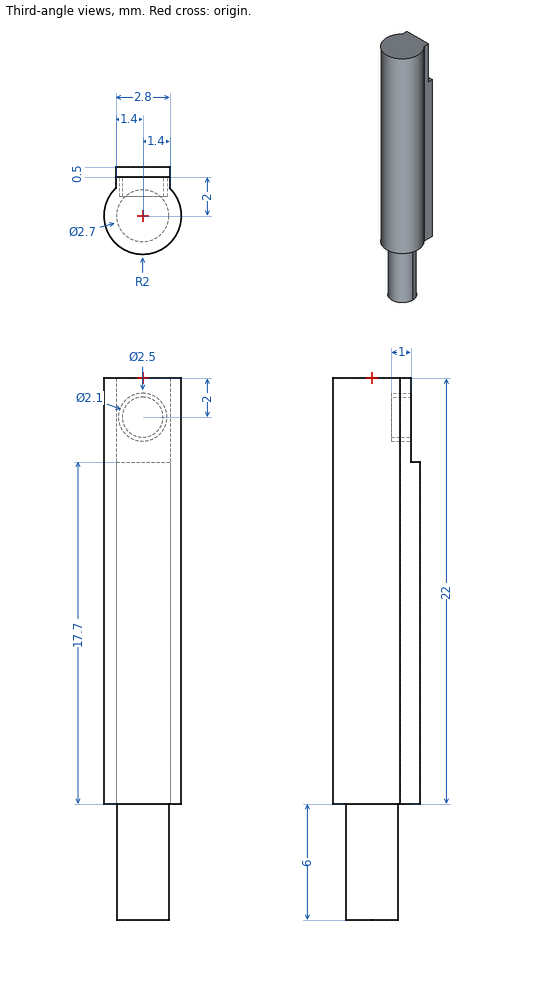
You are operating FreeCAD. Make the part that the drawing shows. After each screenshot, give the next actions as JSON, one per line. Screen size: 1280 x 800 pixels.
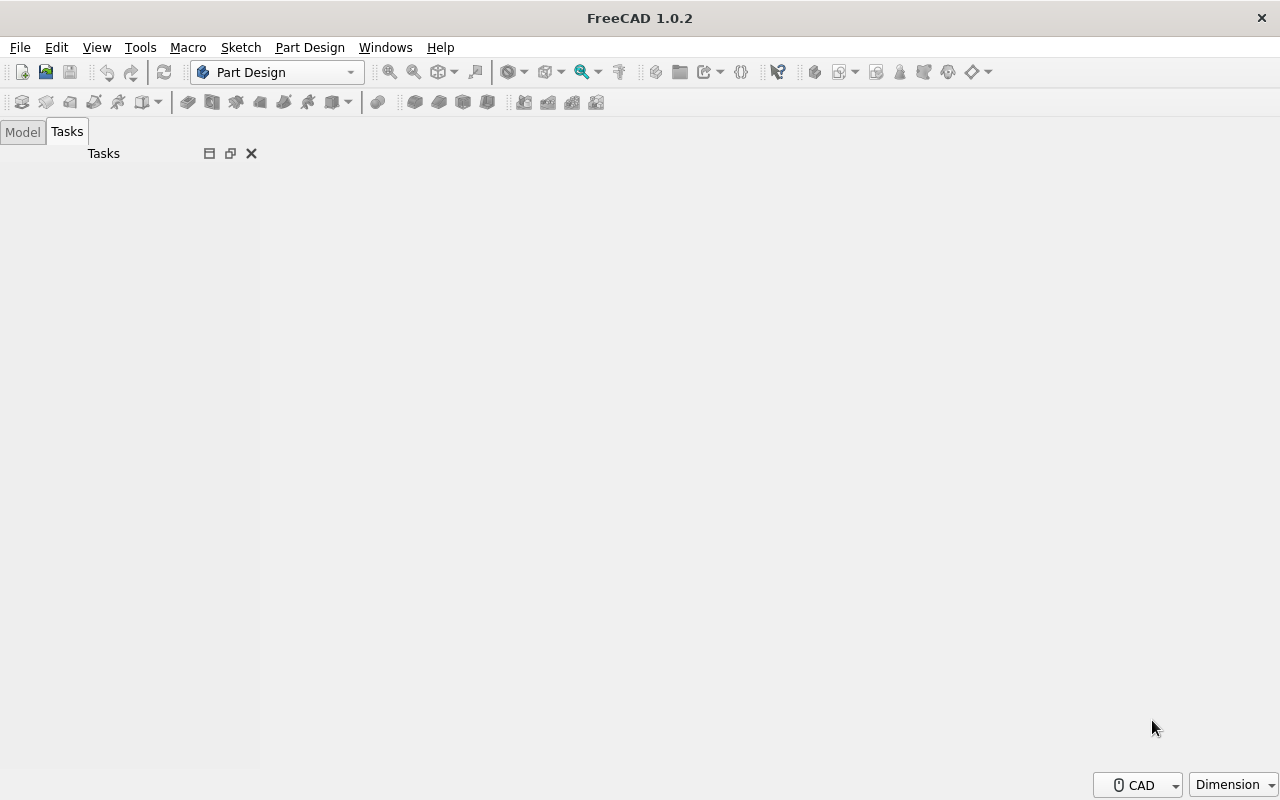
{"action": "key", "text": "ctrl+n"}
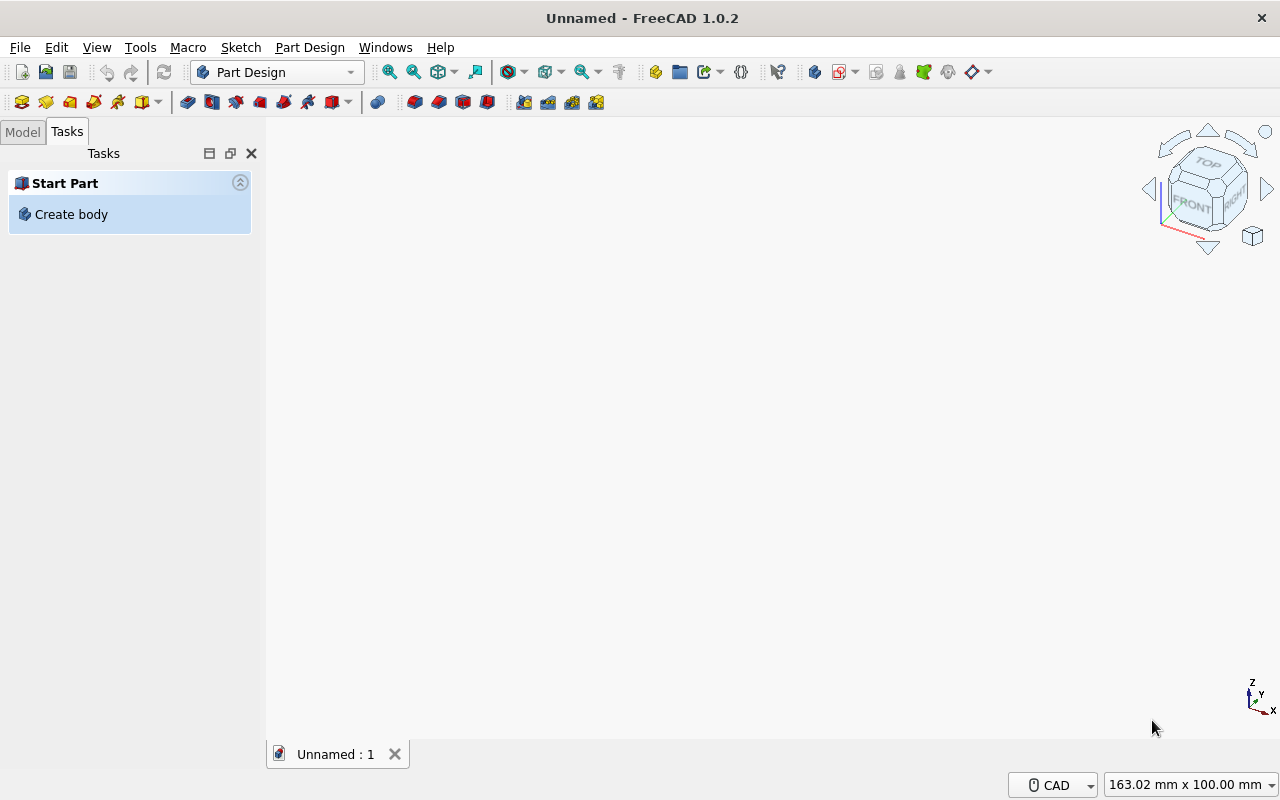
{"action": "left_click", "coordinate": [840, 72]}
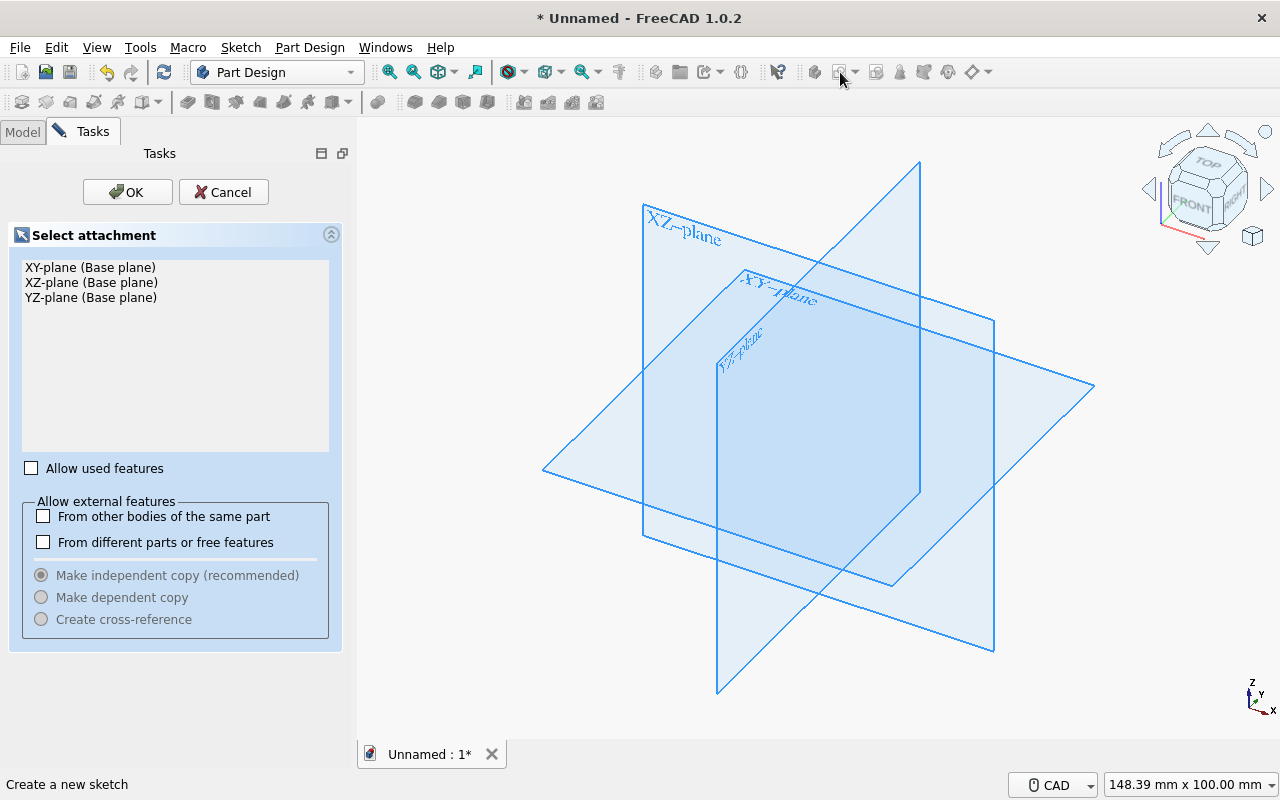
{"action": "left_click", "coordinate": [82, 268]}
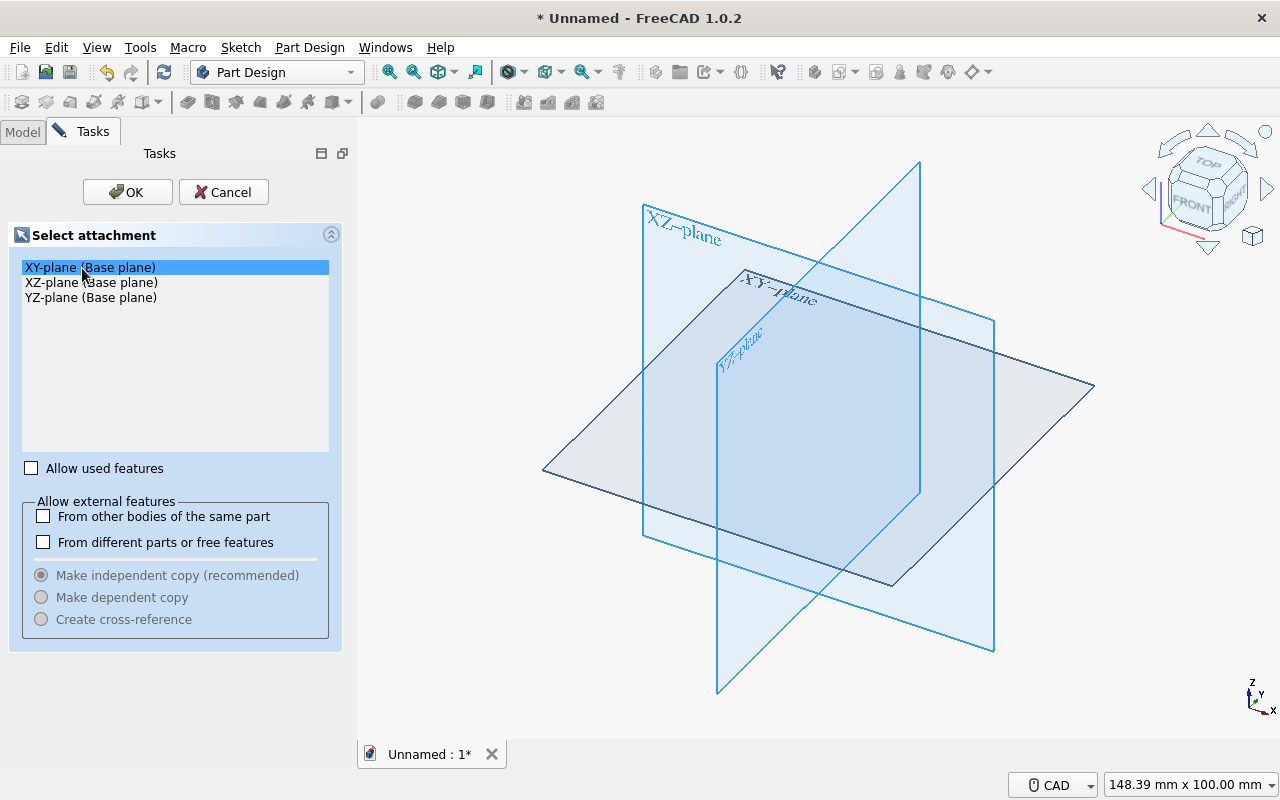
{"action": "left_click", "coordinate": [128, 192]}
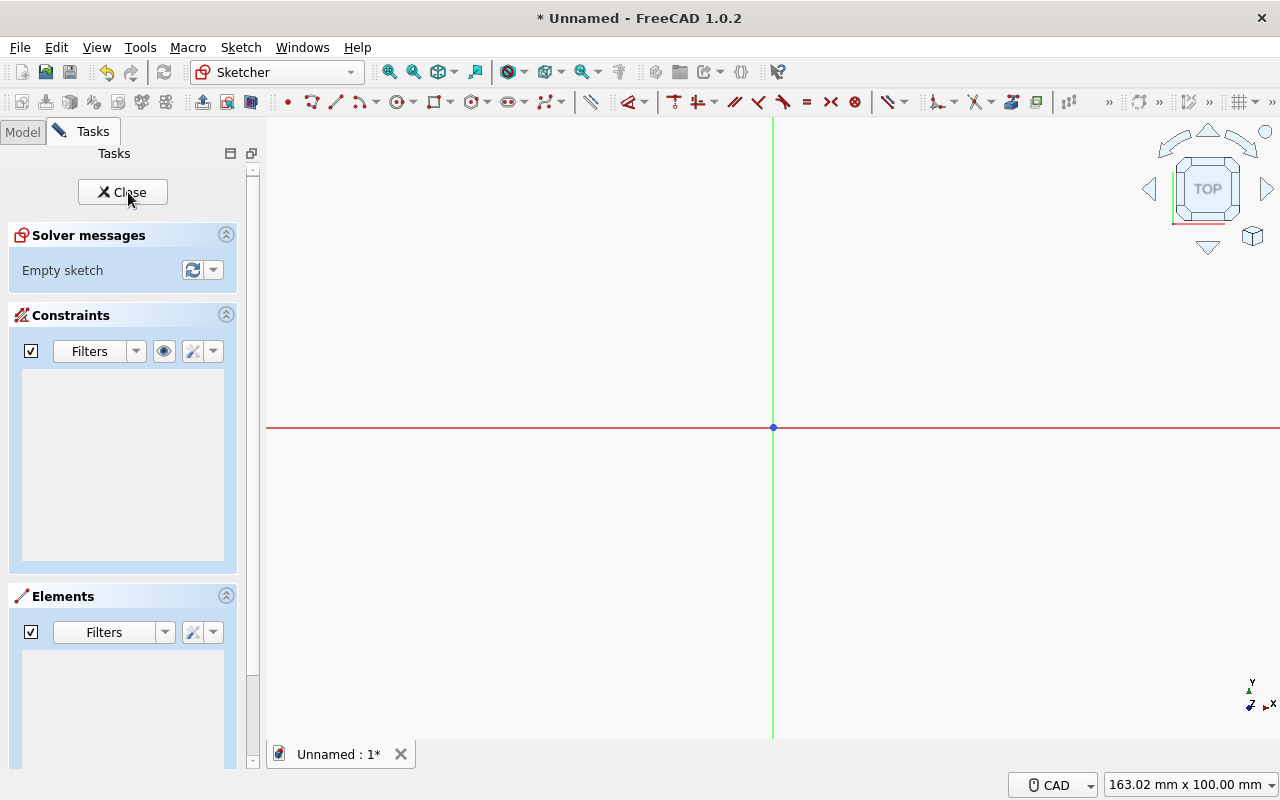
{"action": "scroll", "coordinate": [777, 428], "scroll_direction": "up", "scroll_amount": 14}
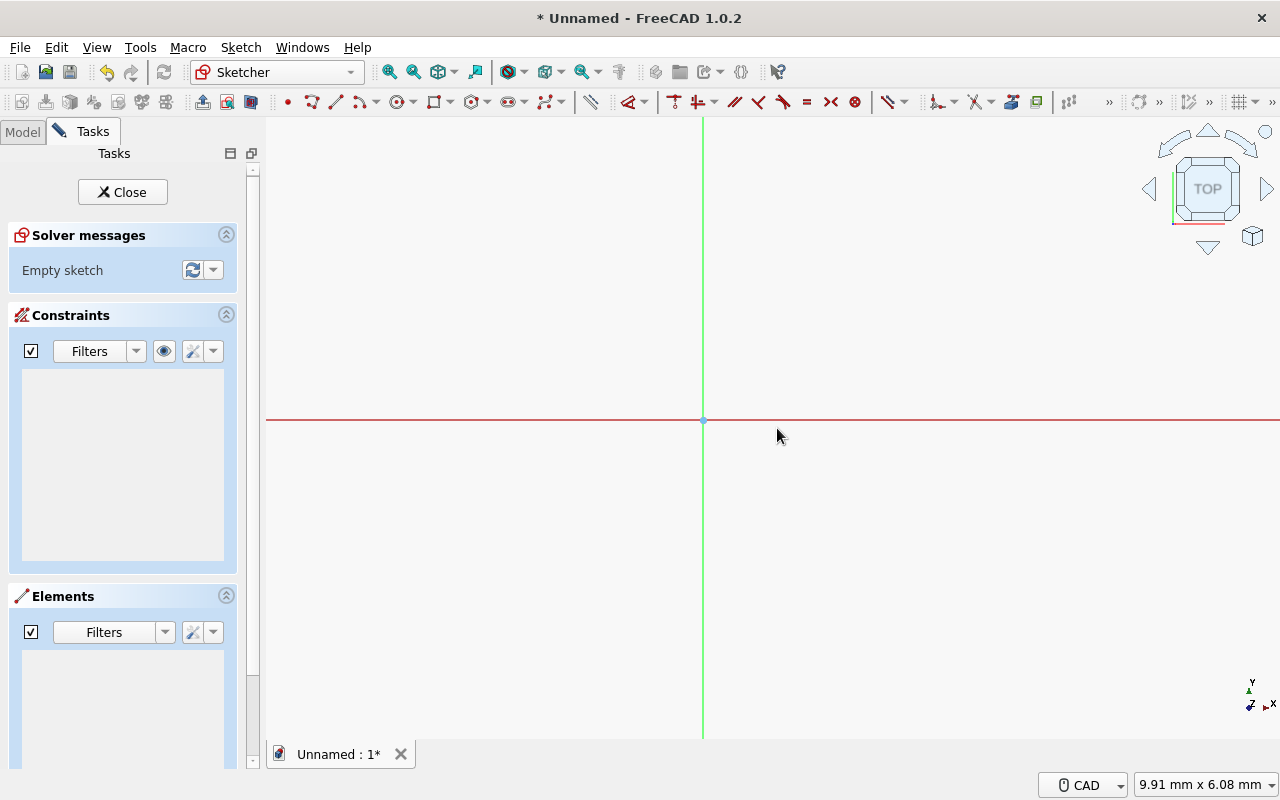
{"action": "left_click", "coordinate": [312, 102]}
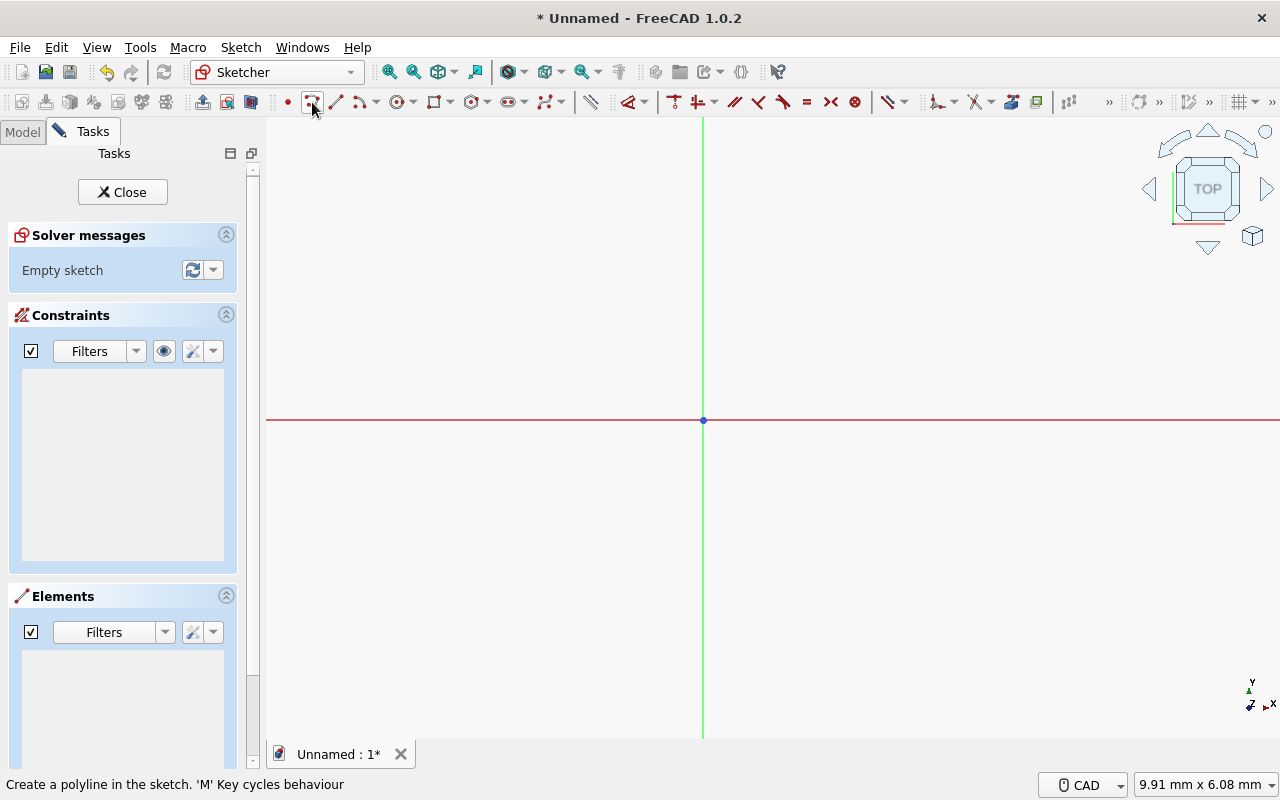
{"action": "left_click", "coordinate": [847, 274]}
{"action": "left_click", "coordinate": [847, 216]}
{"action": "left_click", "coordinate": [560, 216]}
{"action": "left_click", "coordinate": [560, 274]}
{"action": "right_click", "coordinate": [560, 274]}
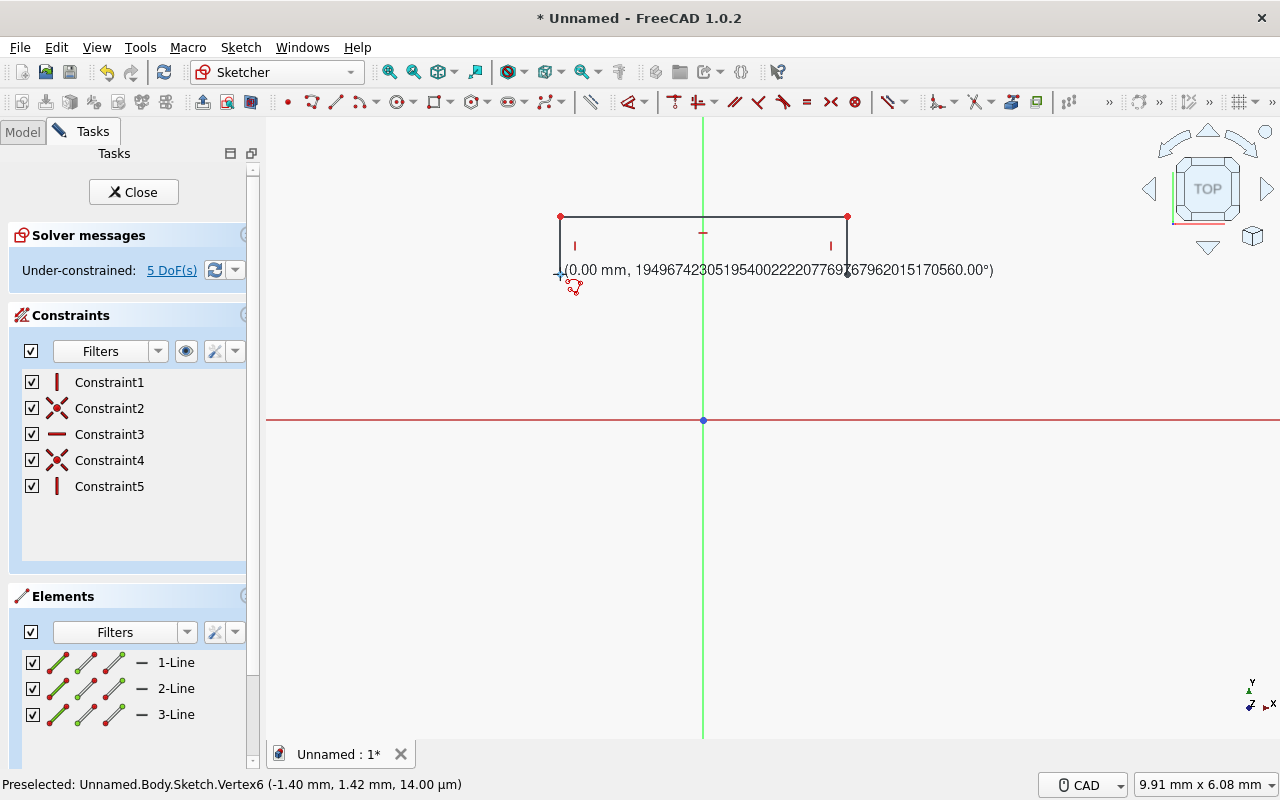
{"action": "left_click", "coordinate": [378, 102]}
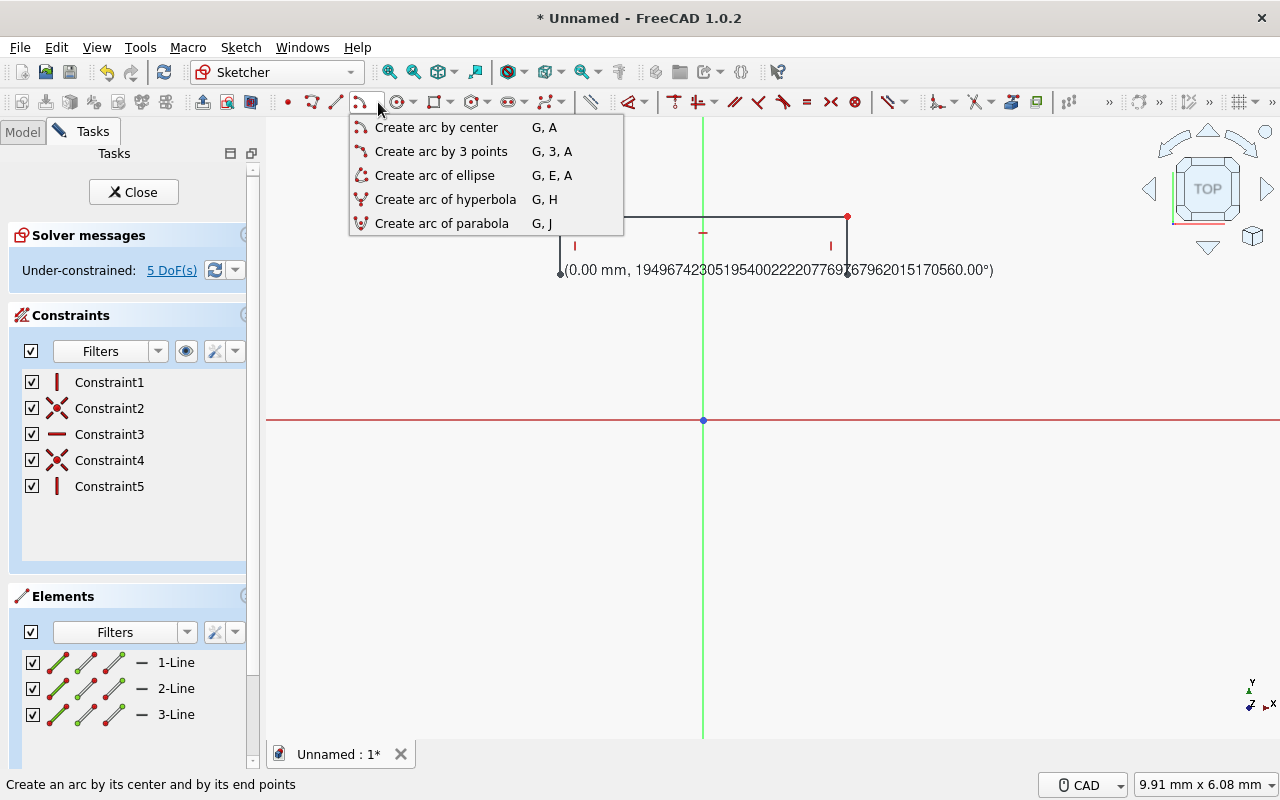
{"action": "left_click", "coordinate": [486, 151]}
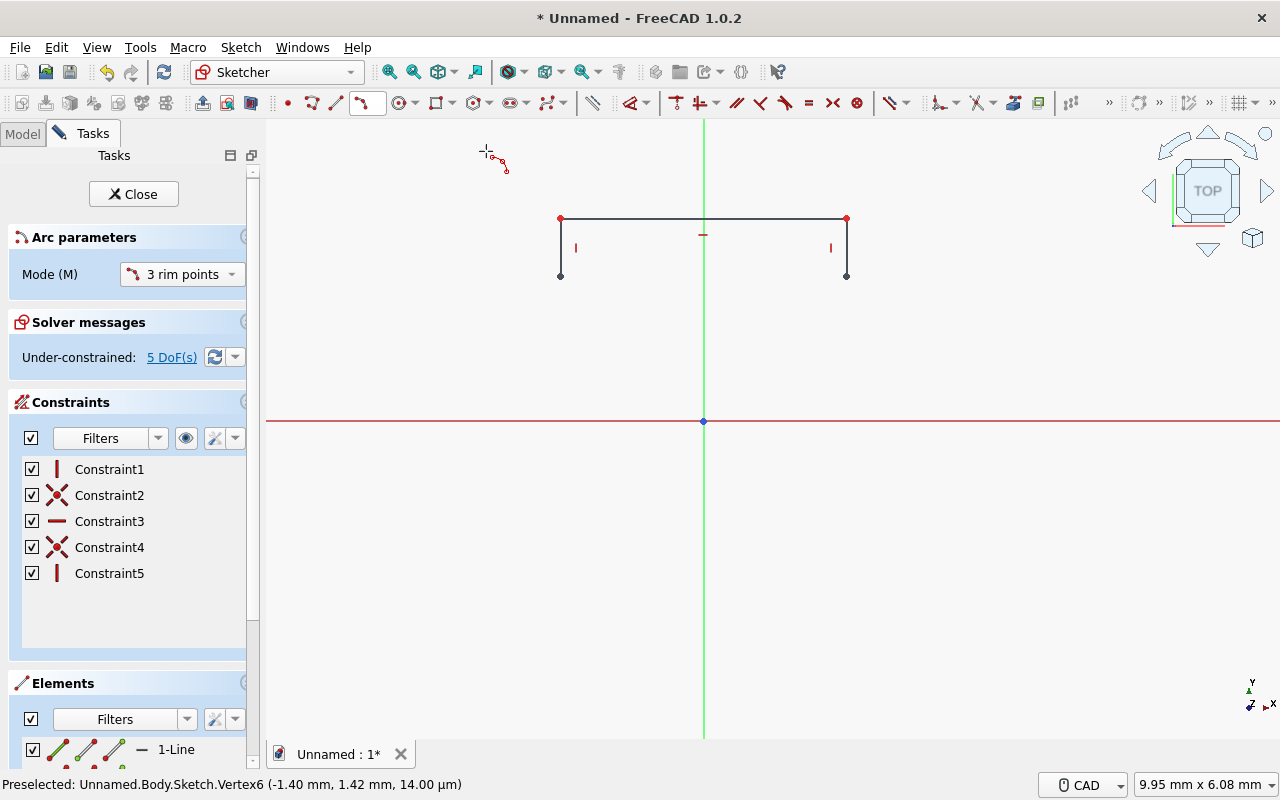
{"action": "left_click", "coordinate": [561, 276]}
{"action": "left_click", "coordinate": [847, 276]}
{"action": "left_click", "coordinate": [611, 603]}
{"action": "key", "text": "Escape"}